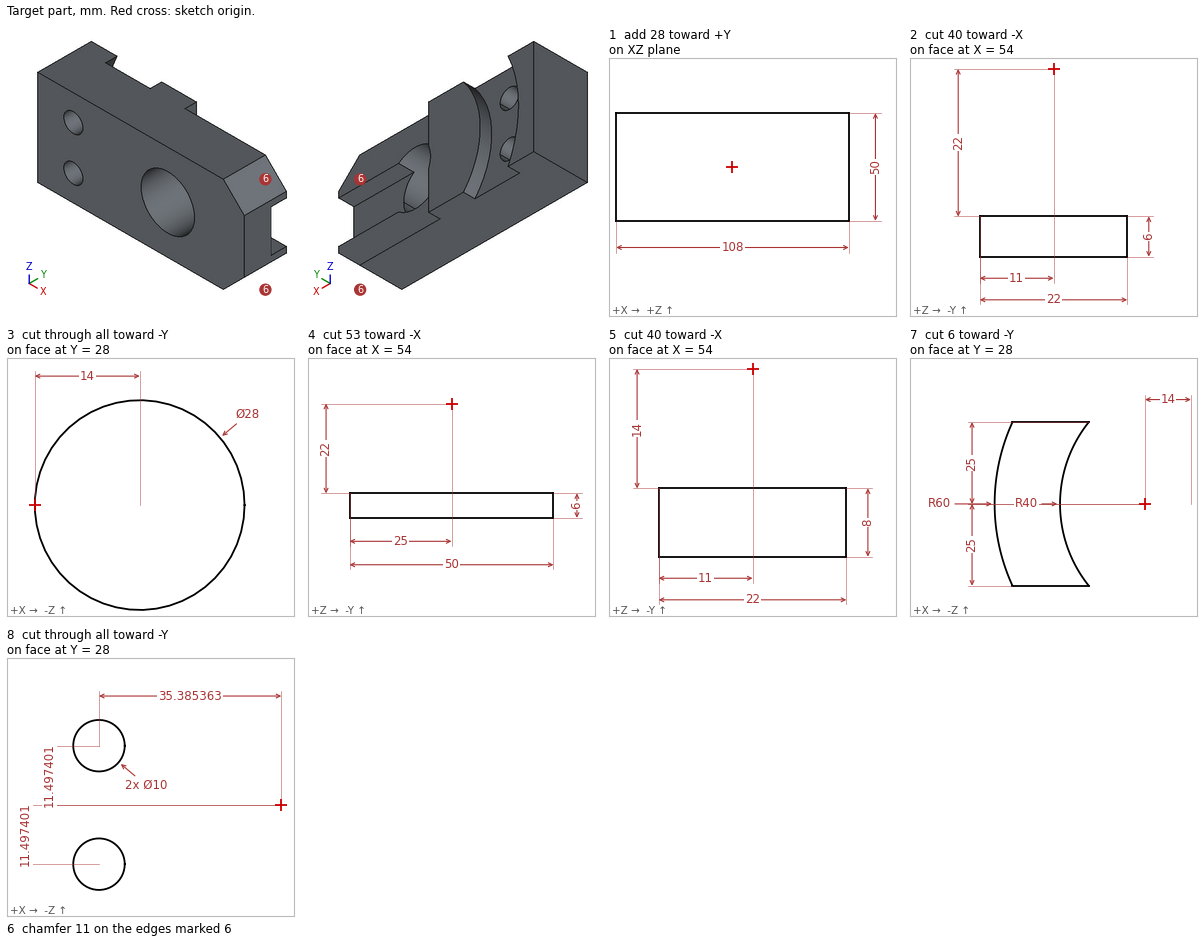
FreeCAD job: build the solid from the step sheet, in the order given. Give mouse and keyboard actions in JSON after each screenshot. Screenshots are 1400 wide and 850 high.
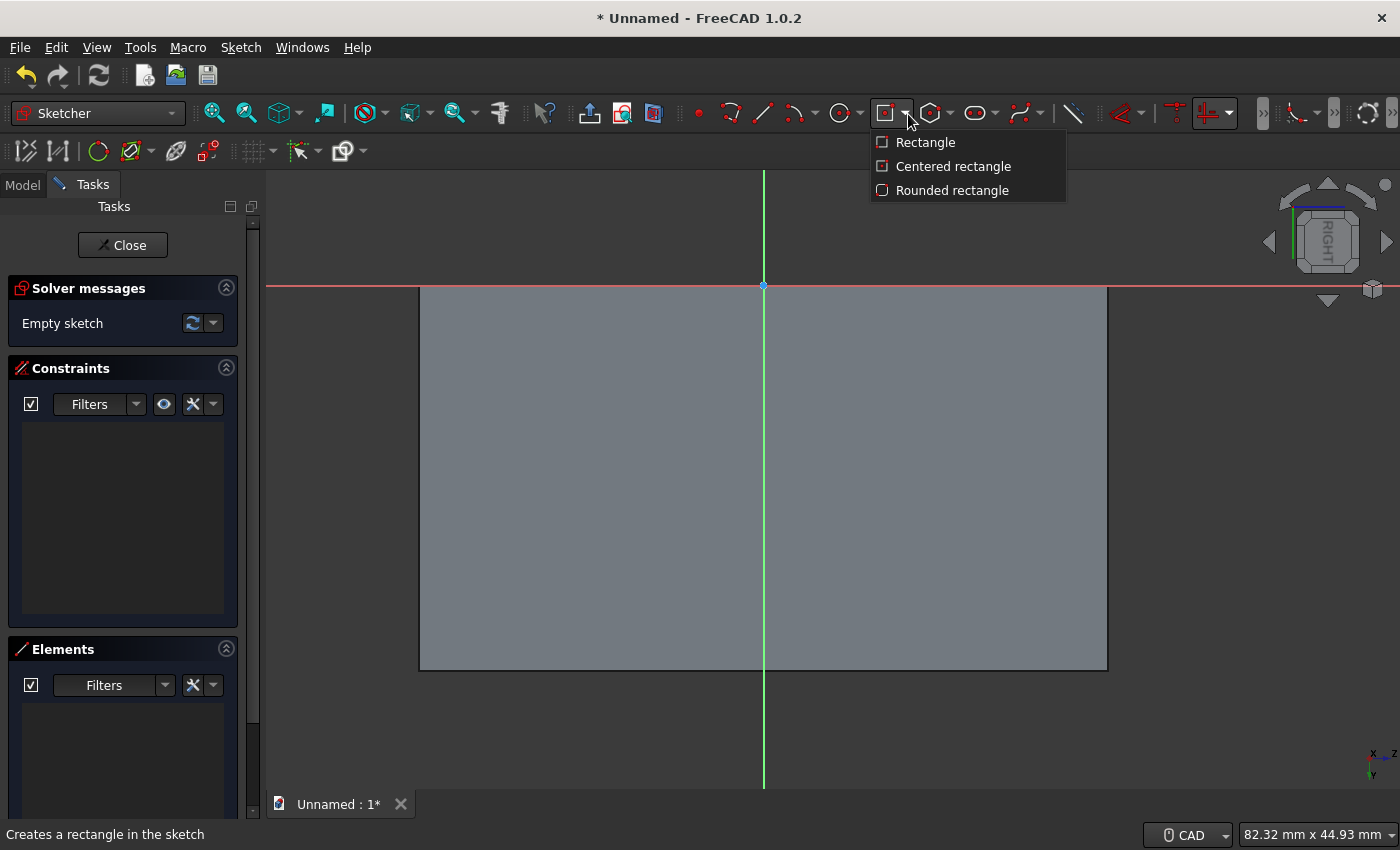
{"action": "left_click", "coordinate": [968, 142]}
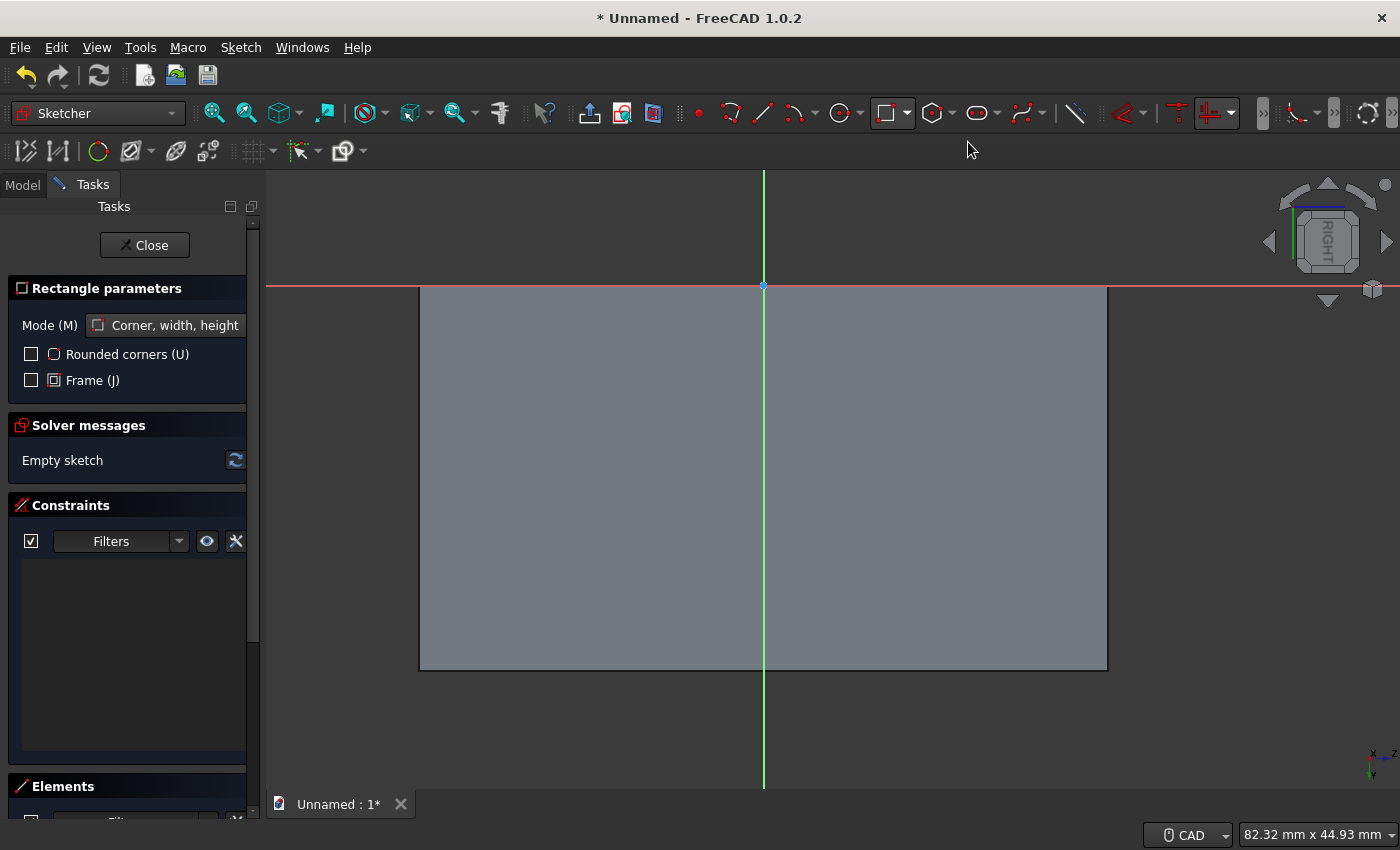
{"action": "left_click", "coordinate": [612, 589]}
{"action": "mouse_move", "coordinate": [915, 671]}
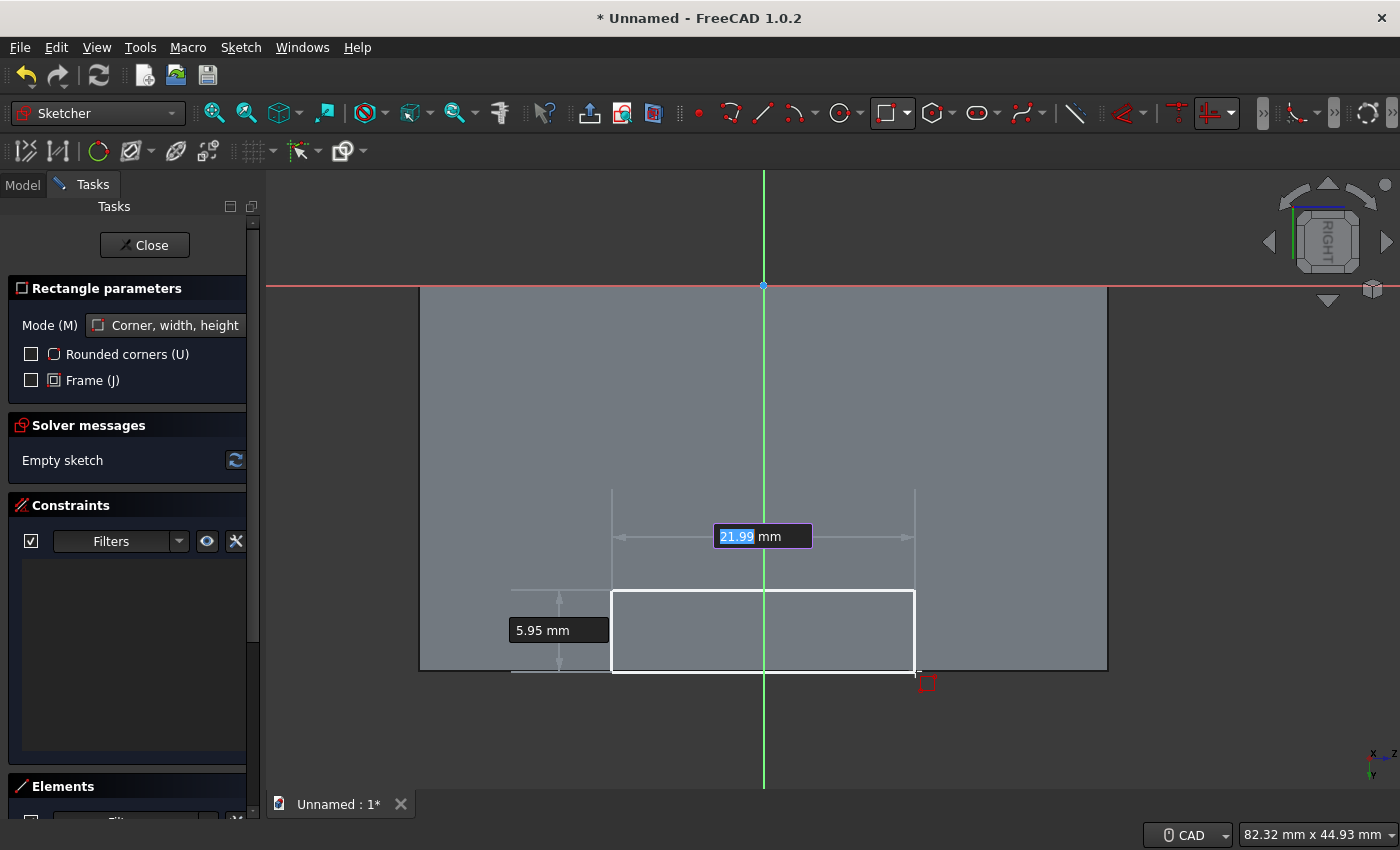
{"action": "type", "text": "22"}
{"action": "key", "text": "Tab"}
{"action": "type", "text": "6"}
{"action": "key", "text": "Return"}
{"action": "key", "text": "Escape"}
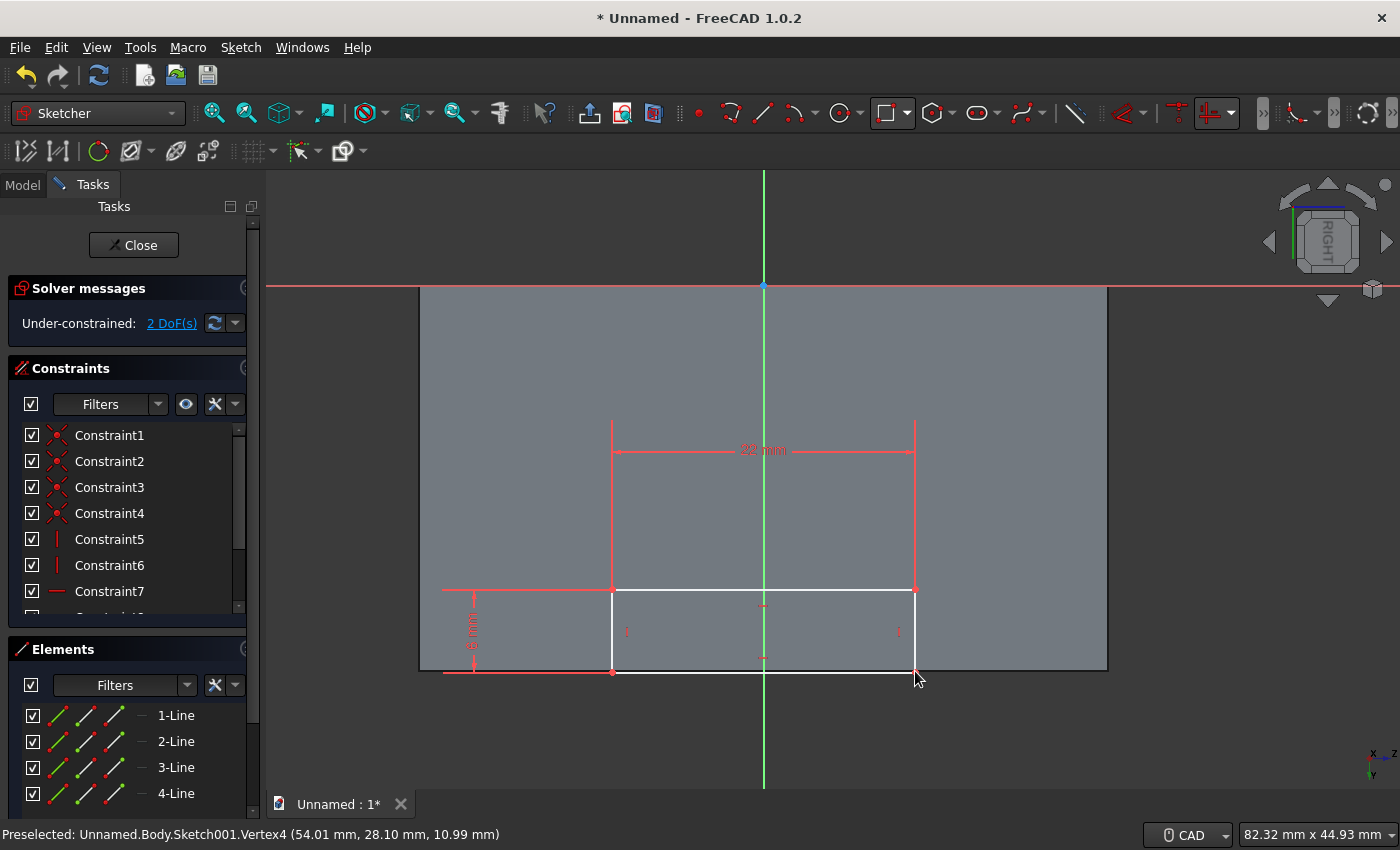
{"action": "key", "text": "d"}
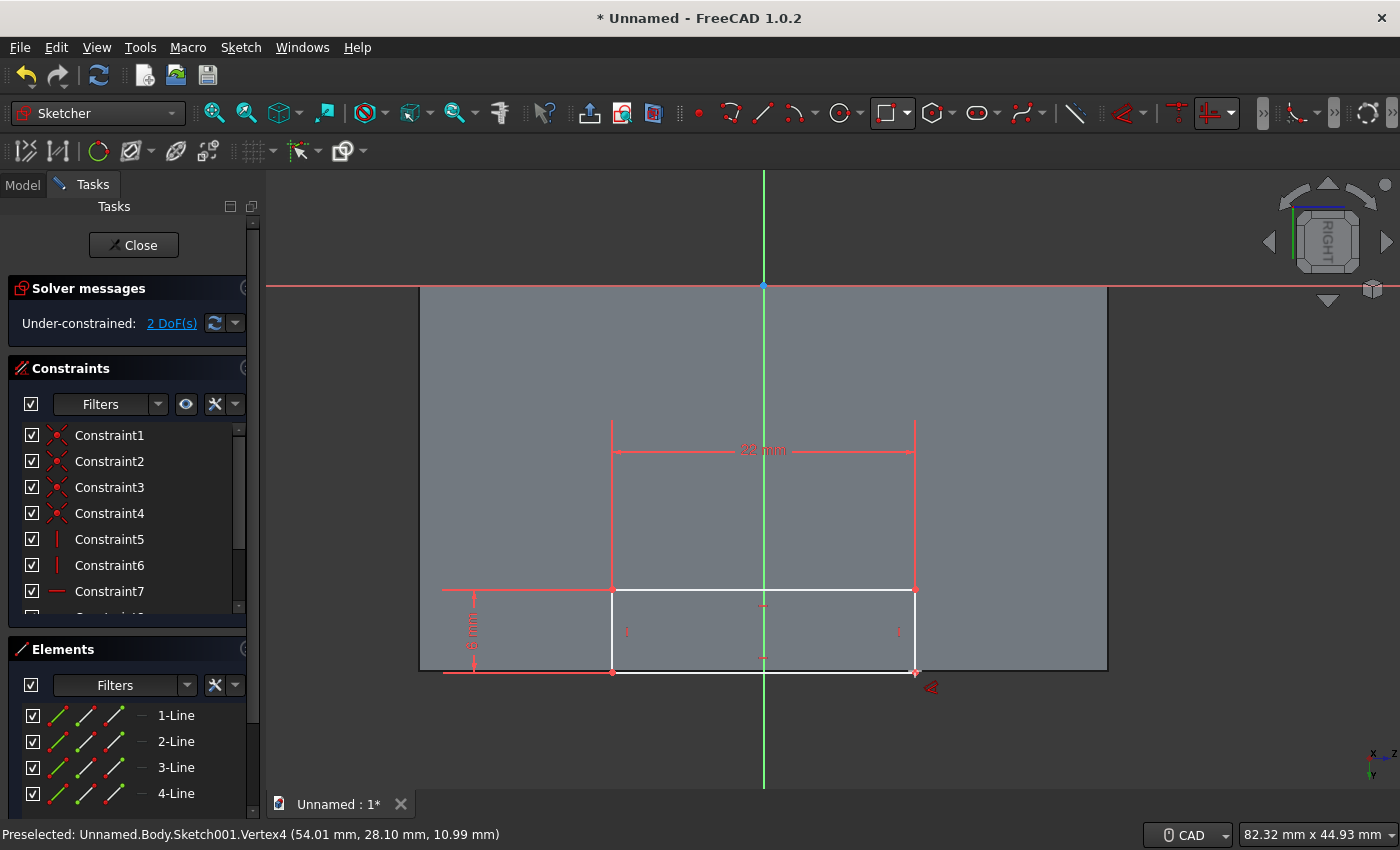
{"action": "left_click", "coordinate": [612, 590]}
{"action": "left_click", "coordinate": [688, 252]}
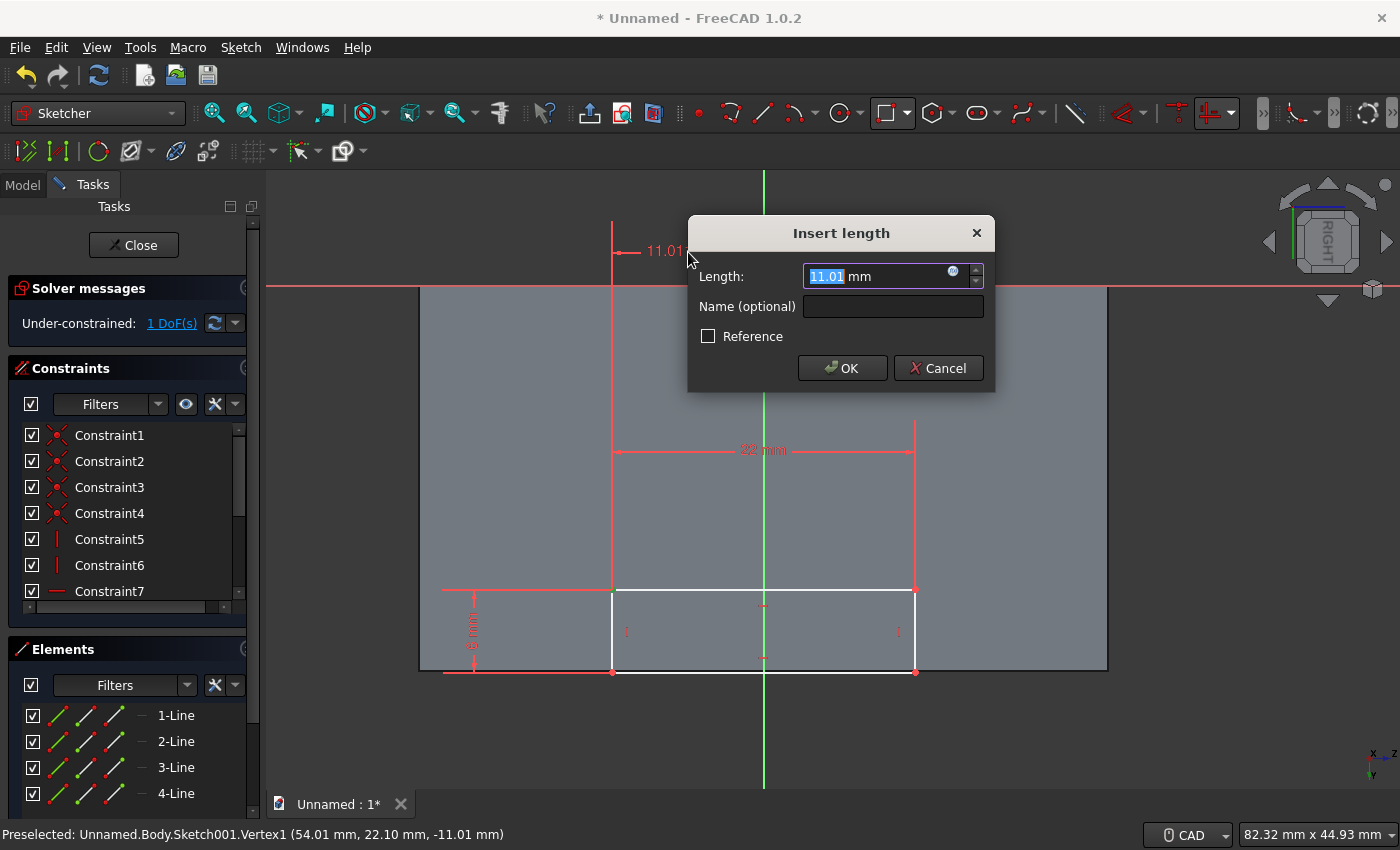
{"action": "type", "text": "11"}
{"action": "key", "text": "Return"}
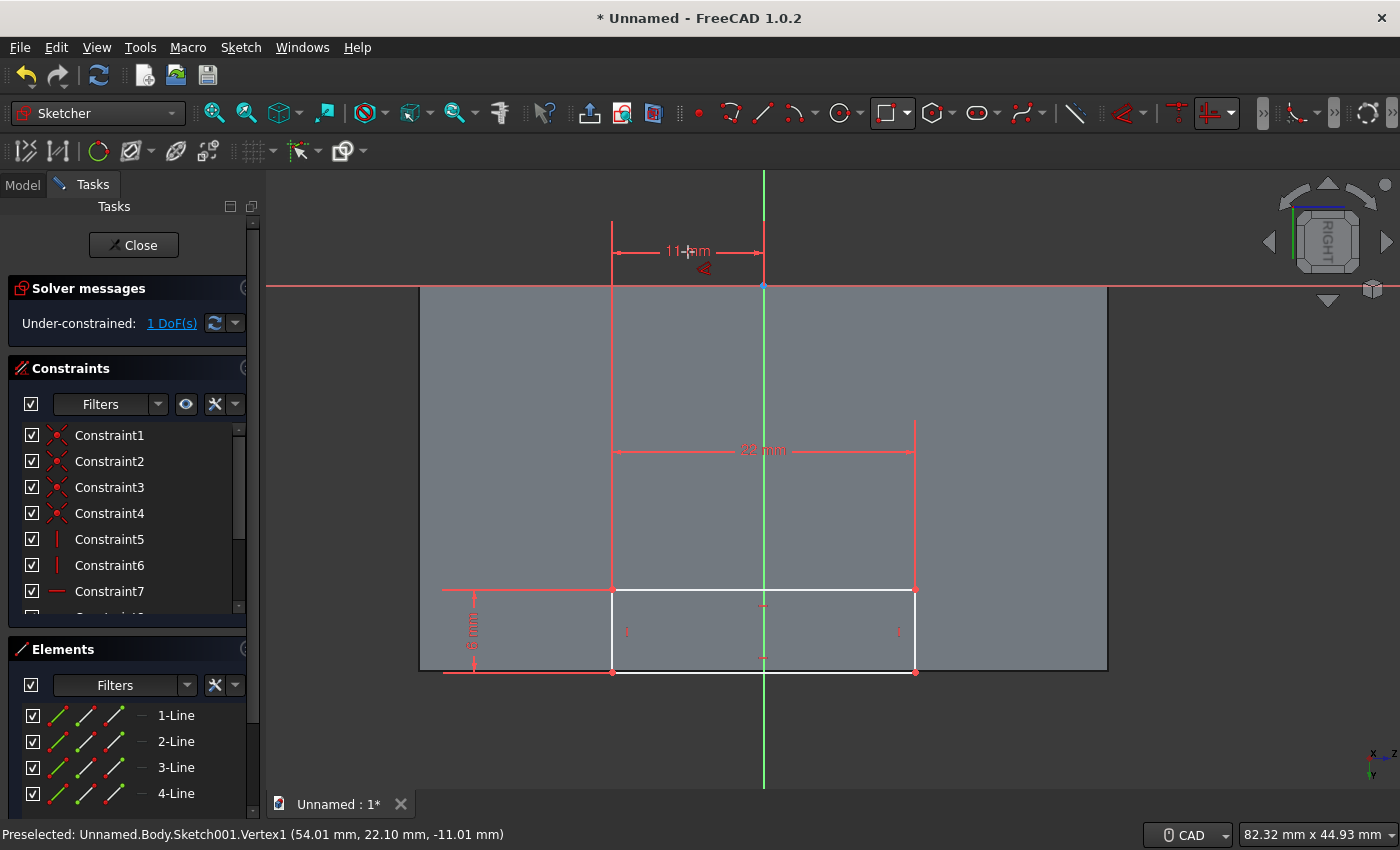
{"action": "left_click", "coordinate": [612, 590]}
{"action": "left_click", "coordinate": [578, 438]}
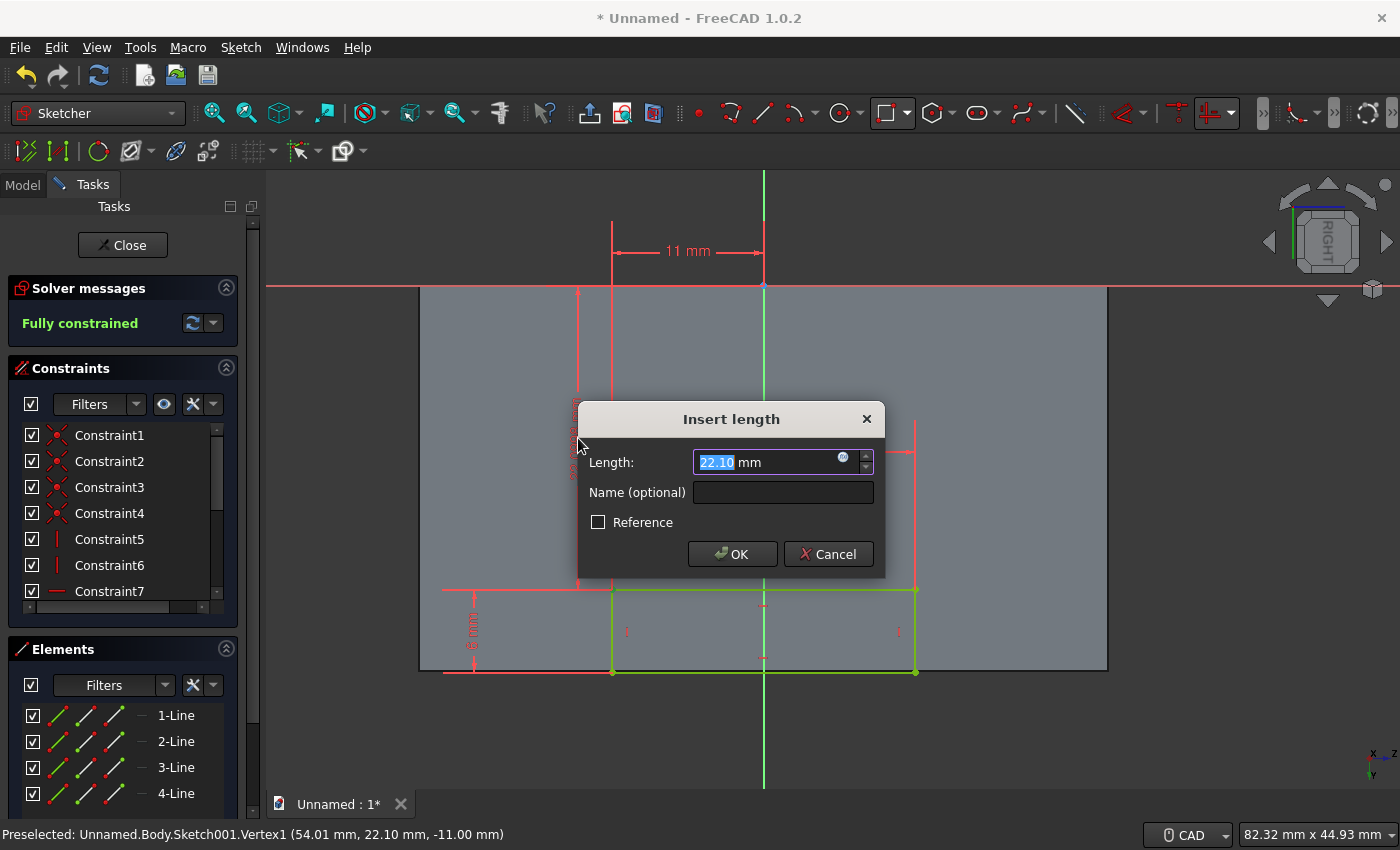
{"action": "type", "text": "22"}
{"action": "key", "text": "Return"}
{"action": "key", "text": "Escape"}